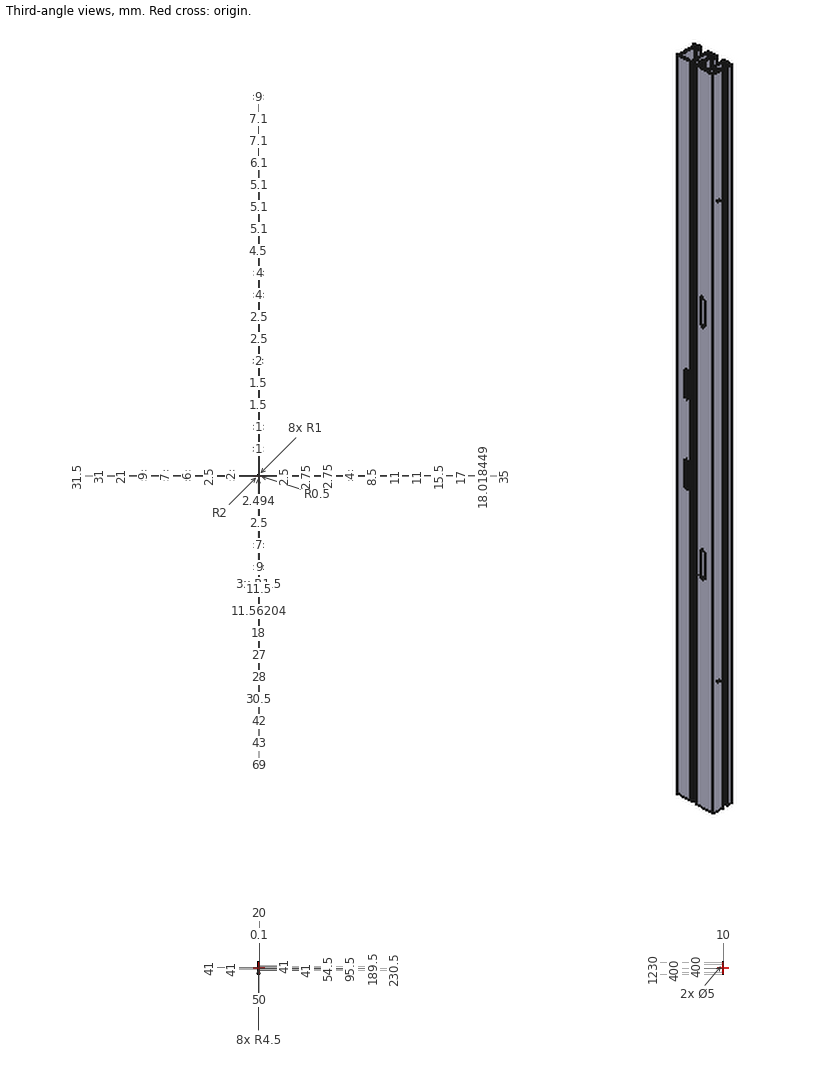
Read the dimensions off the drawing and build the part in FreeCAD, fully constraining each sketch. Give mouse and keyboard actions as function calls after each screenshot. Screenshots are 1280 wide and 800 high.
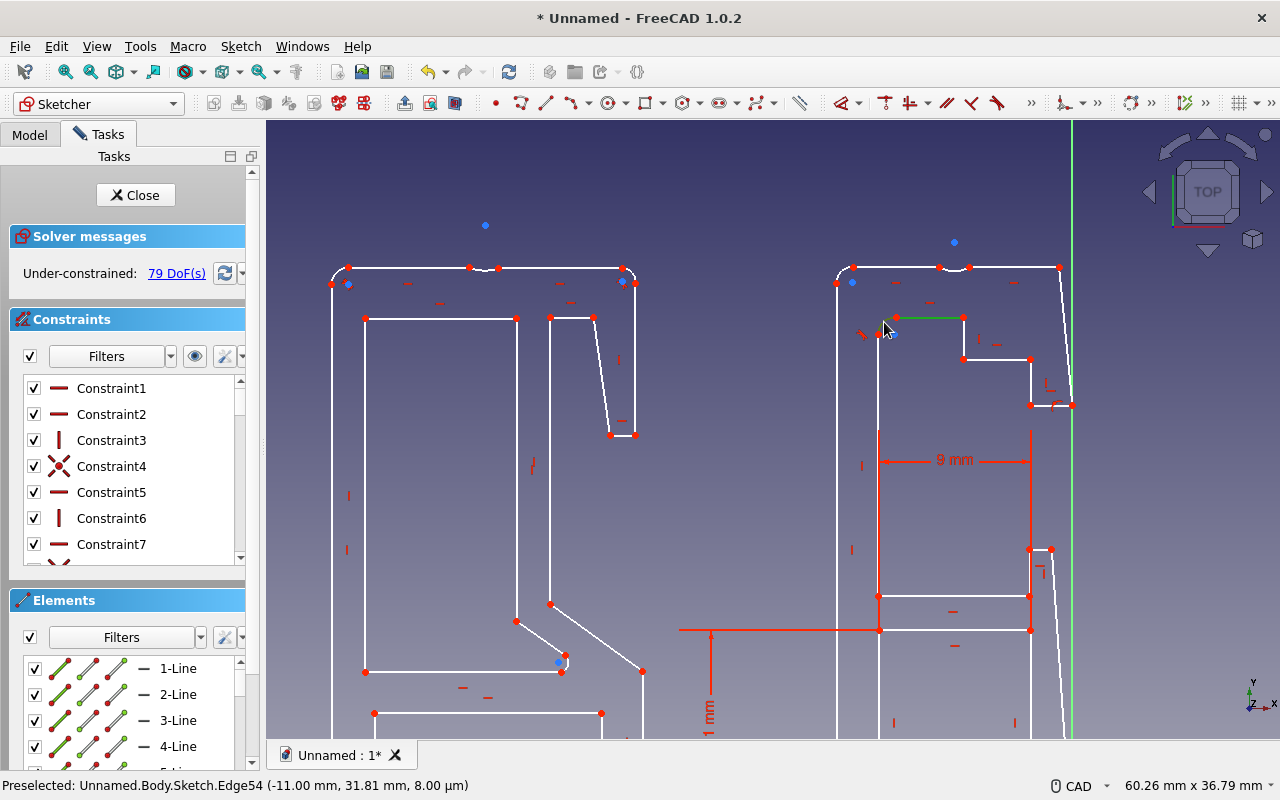
click(997, 104)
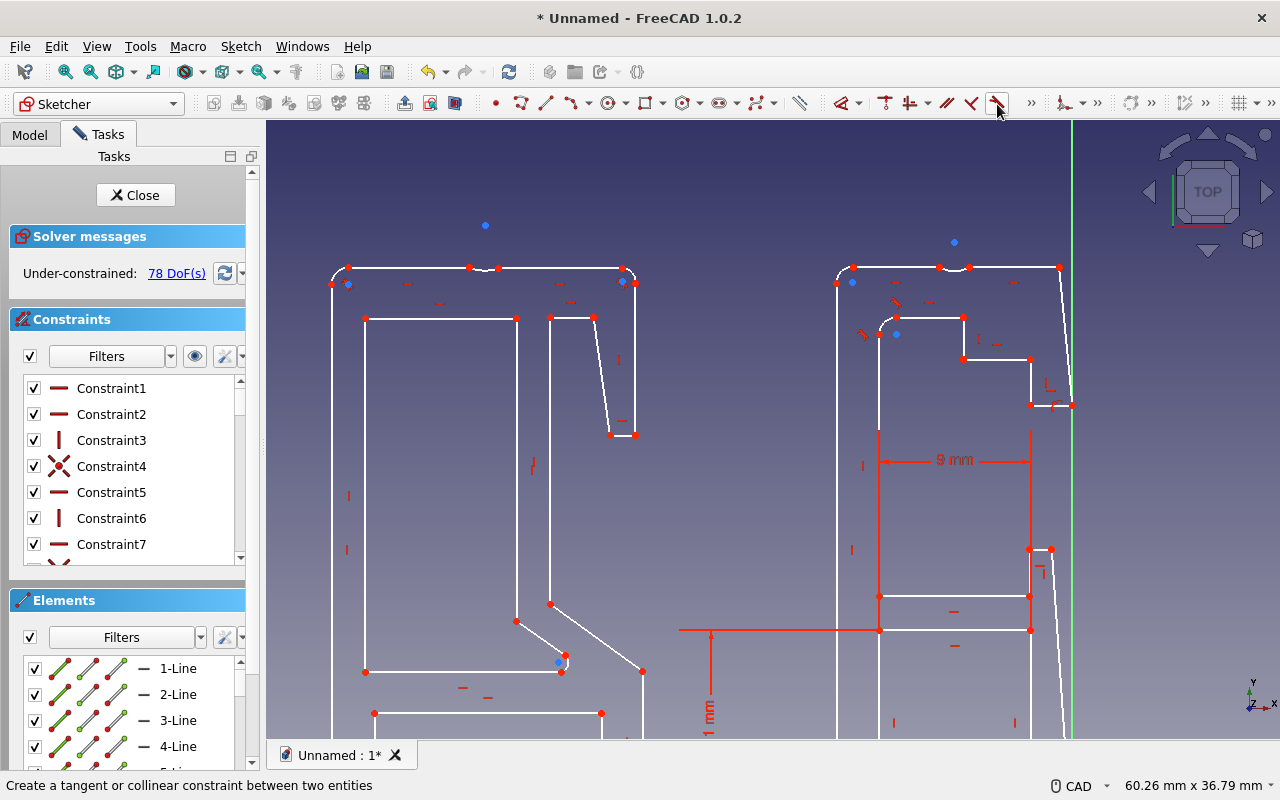
click(914, 267)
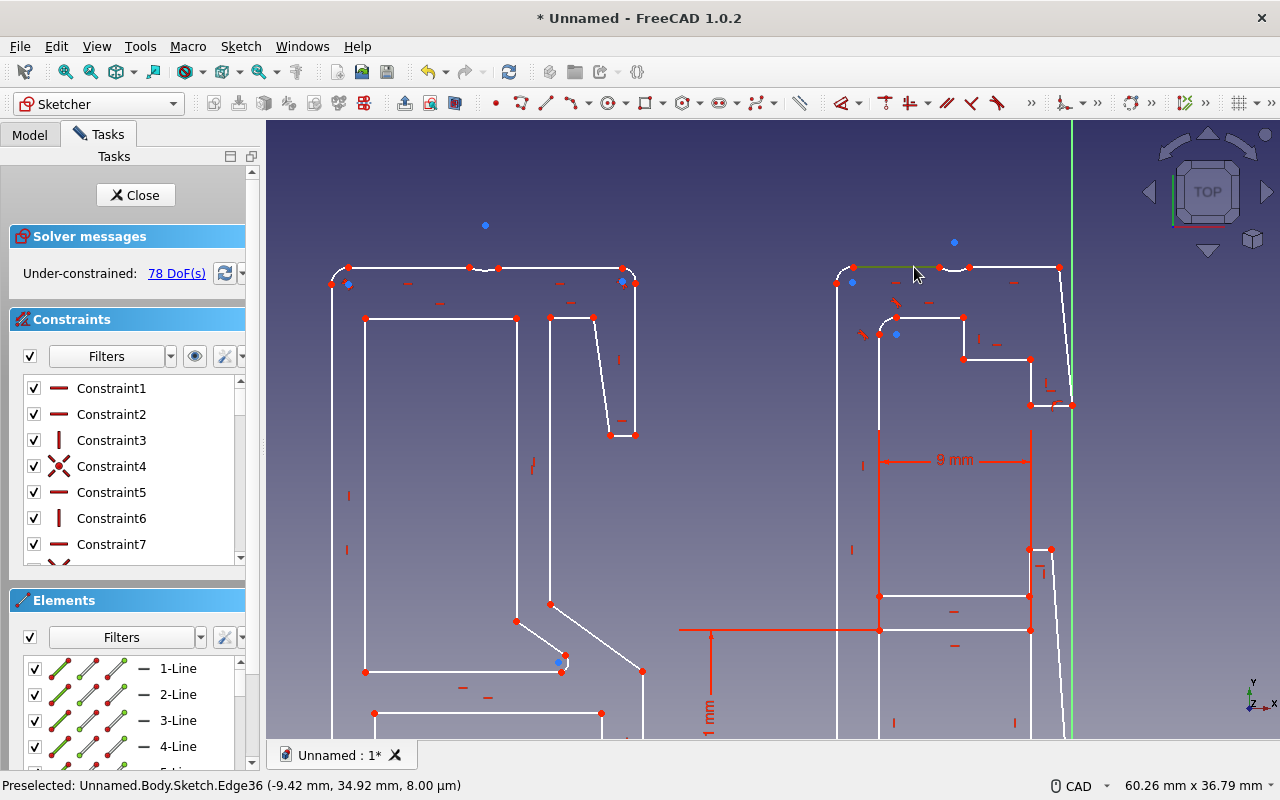
click(841, 272)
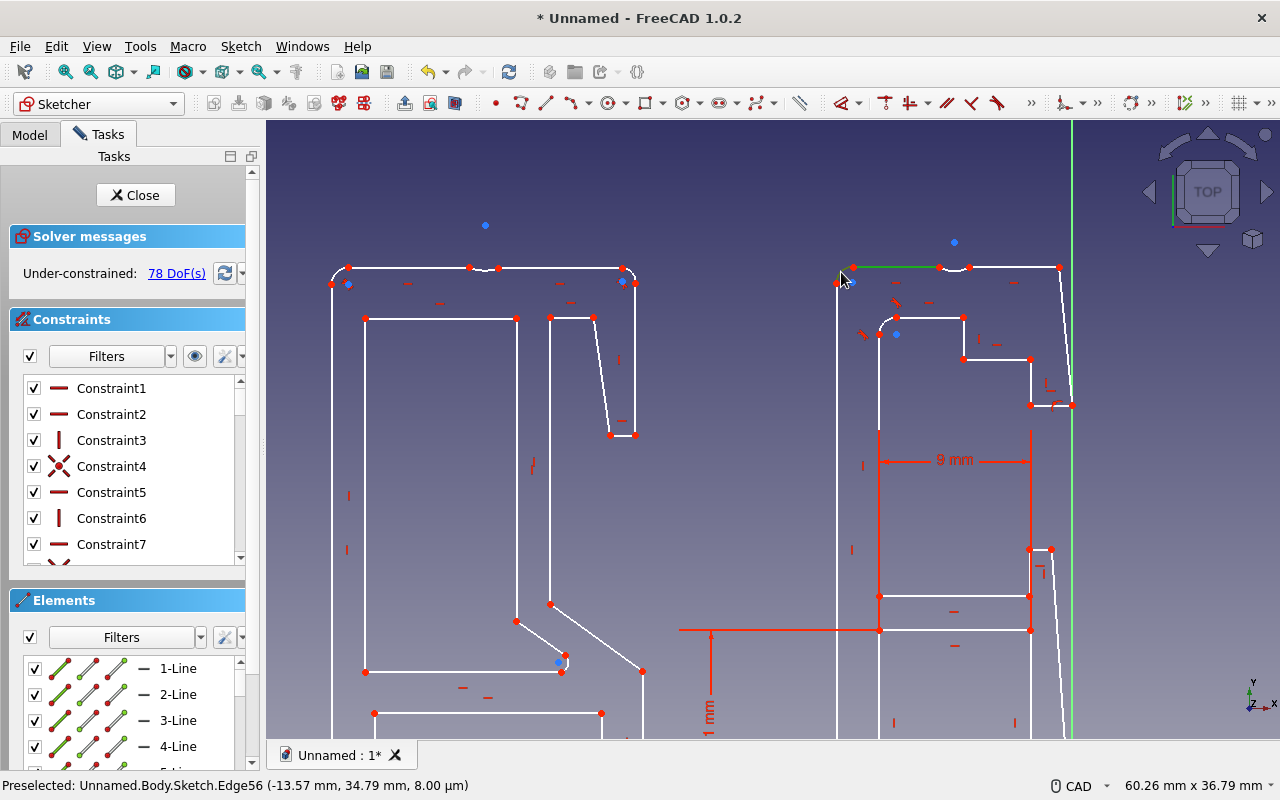
click(997, 104)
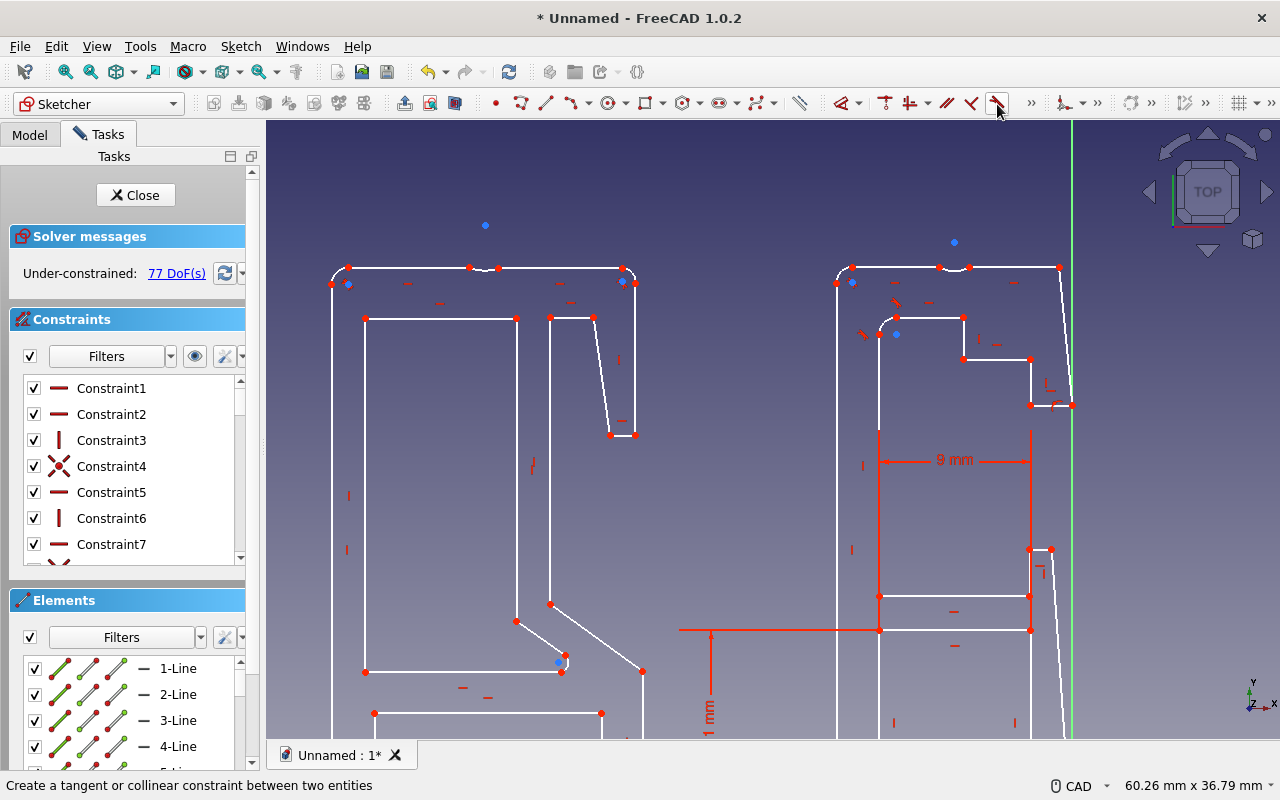
click(837, 443)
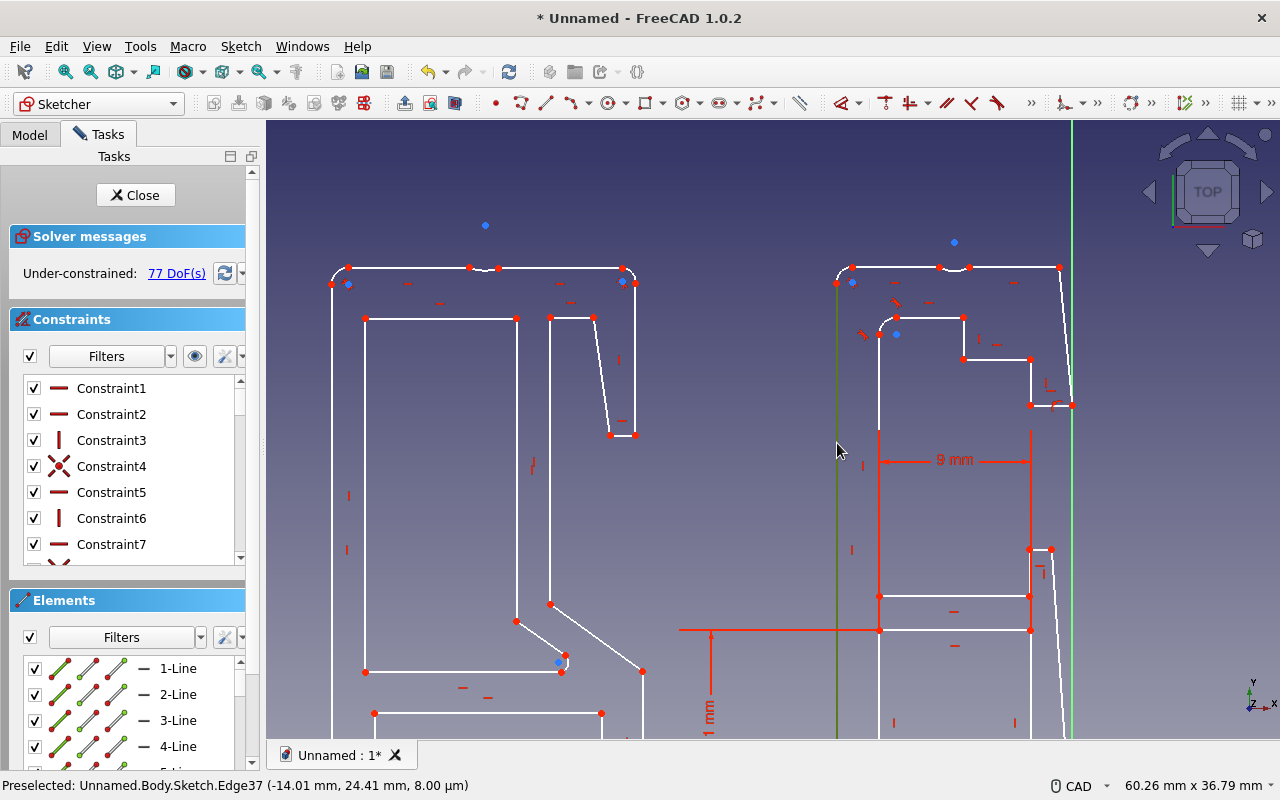
click(841, 272)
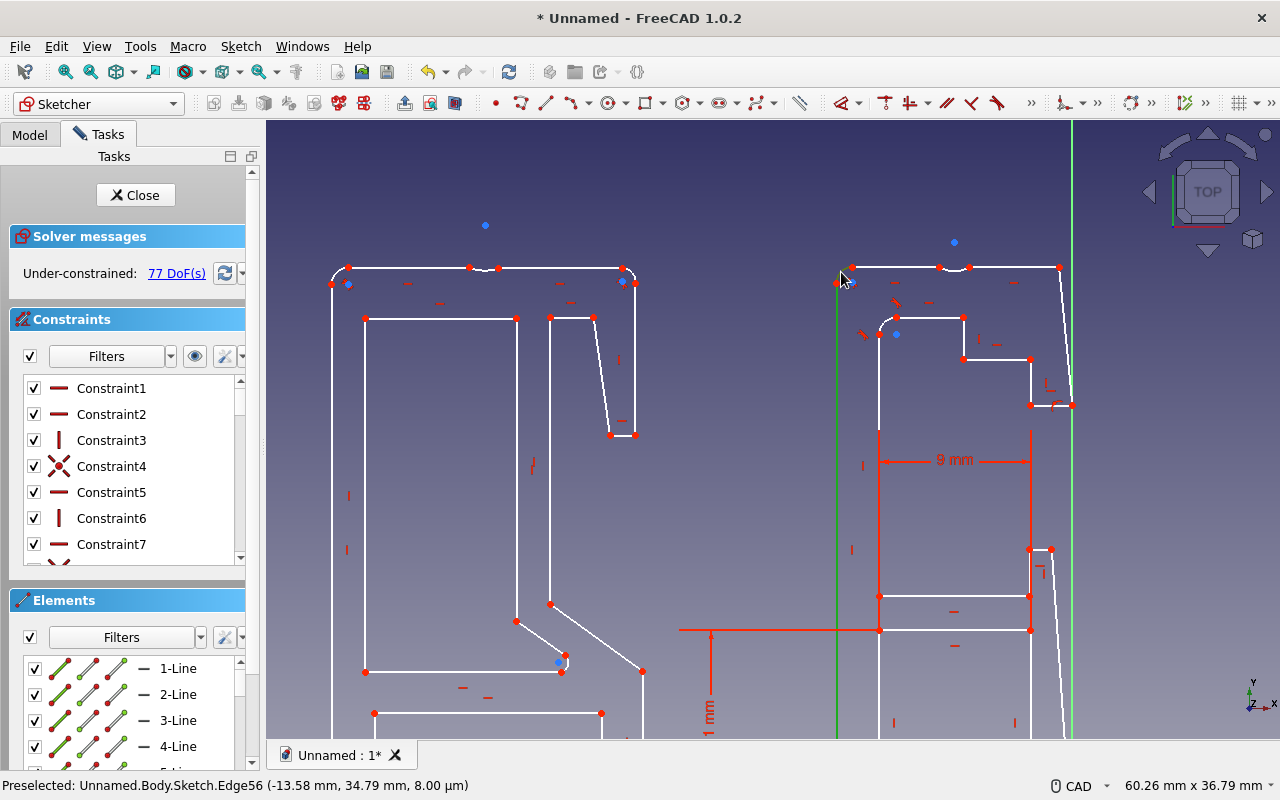
click(997, 104)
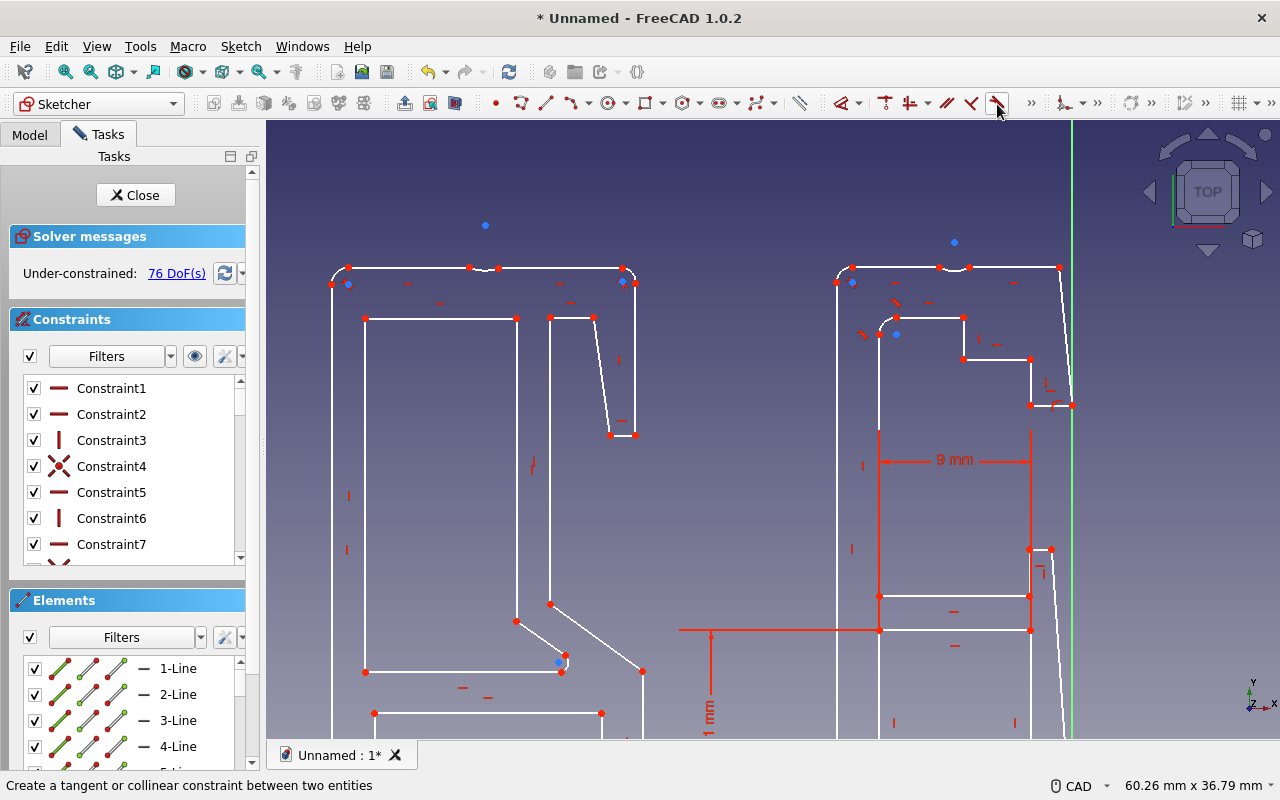
click(635, 390)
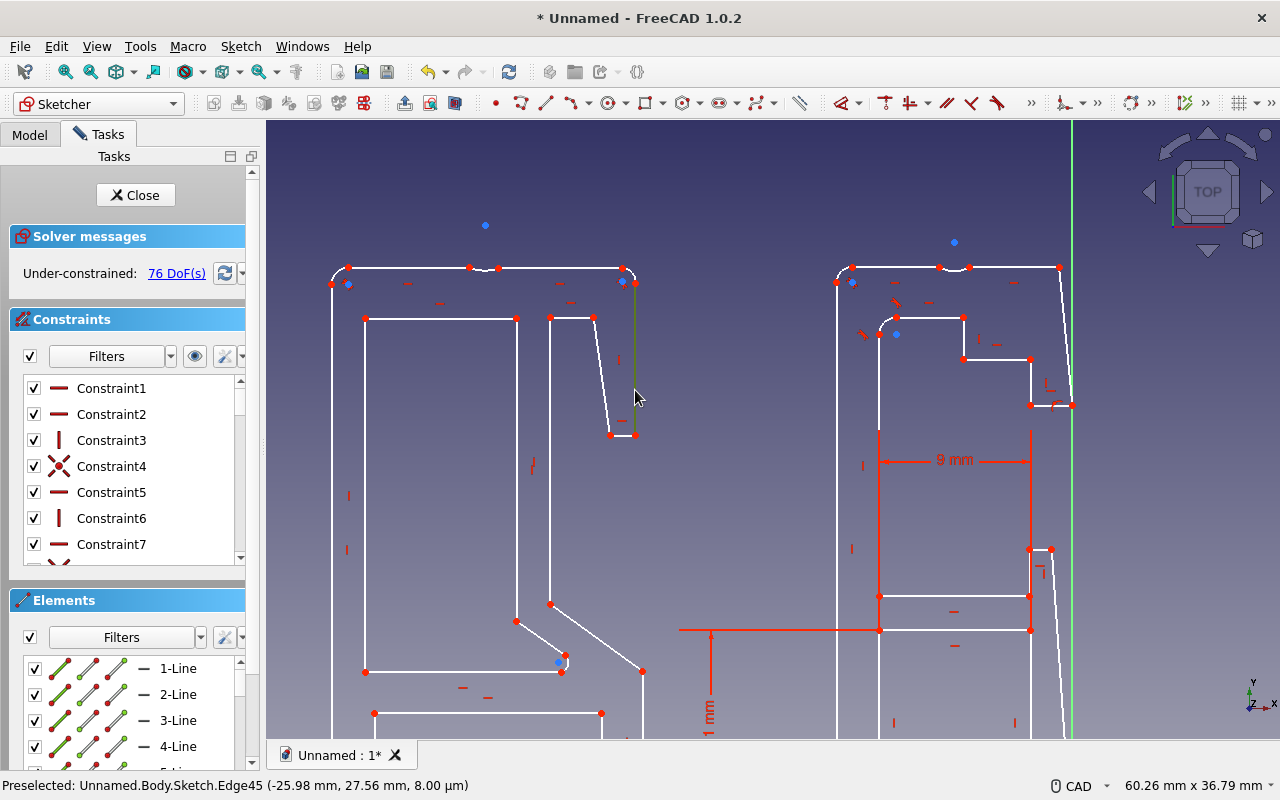
scroll(632, 273, up, 2)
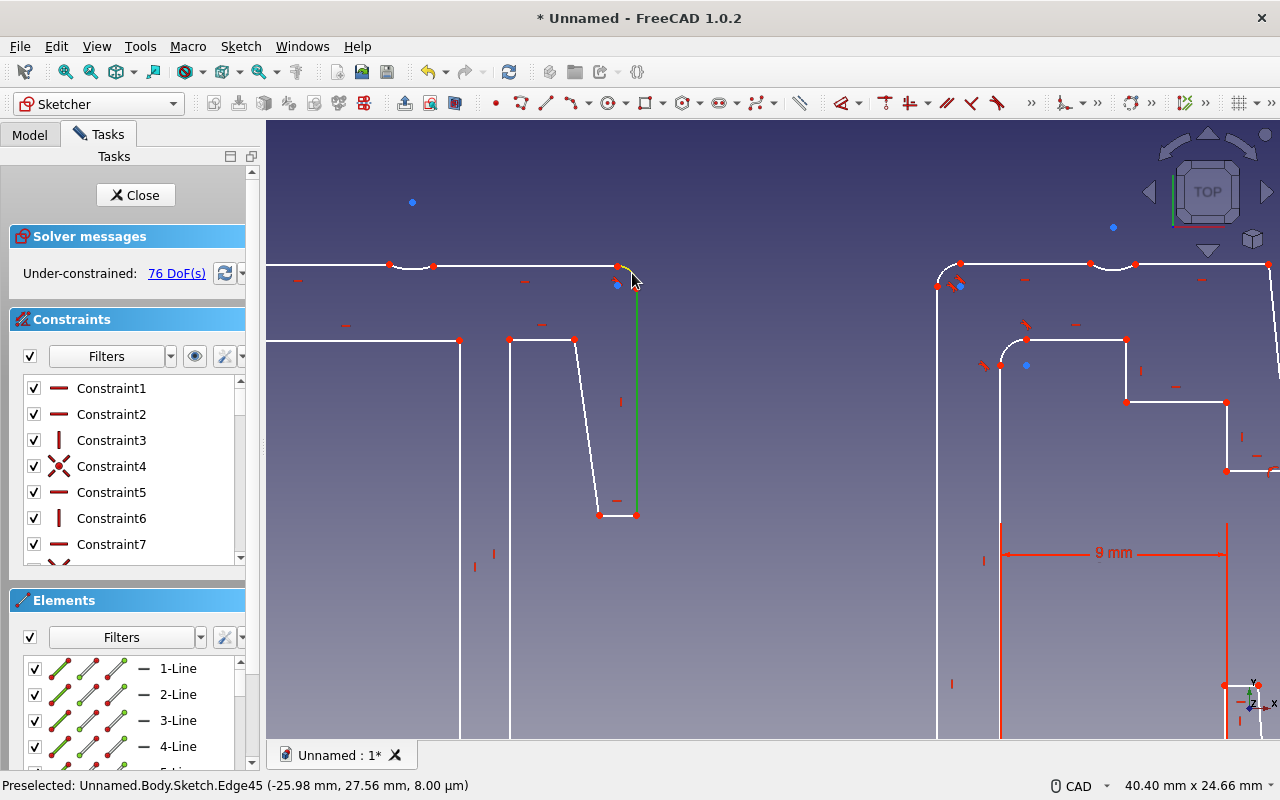
click(632, 273)